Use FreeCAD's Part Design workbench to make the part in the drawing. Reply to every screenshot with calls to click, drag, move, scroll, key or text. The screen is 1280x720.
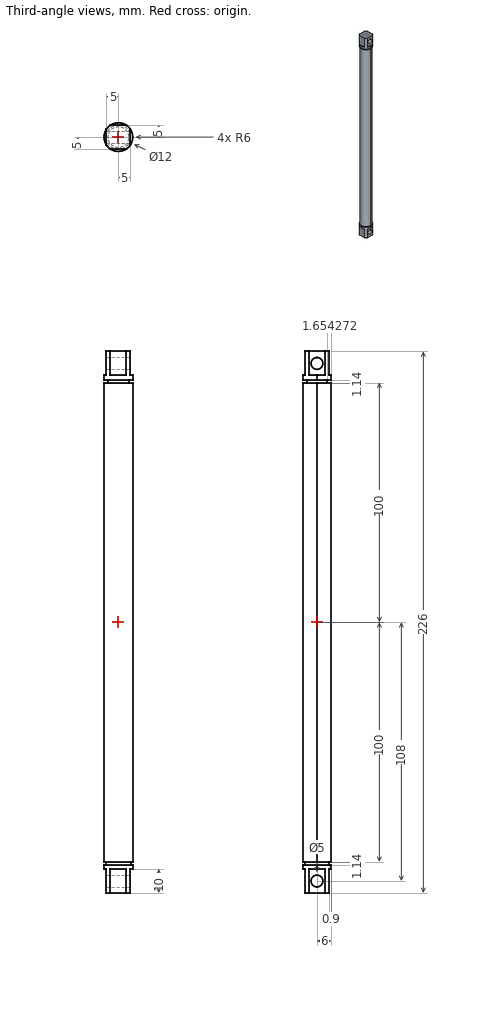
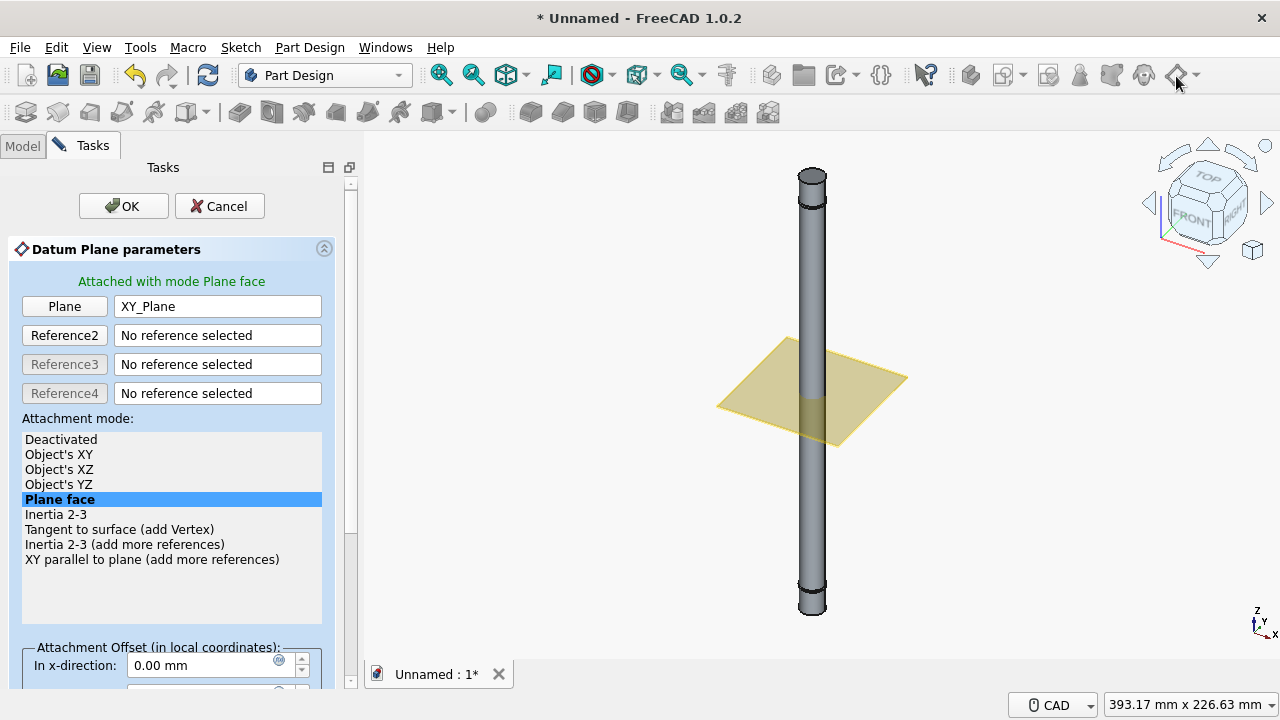
scroll(351, 432, down, 2)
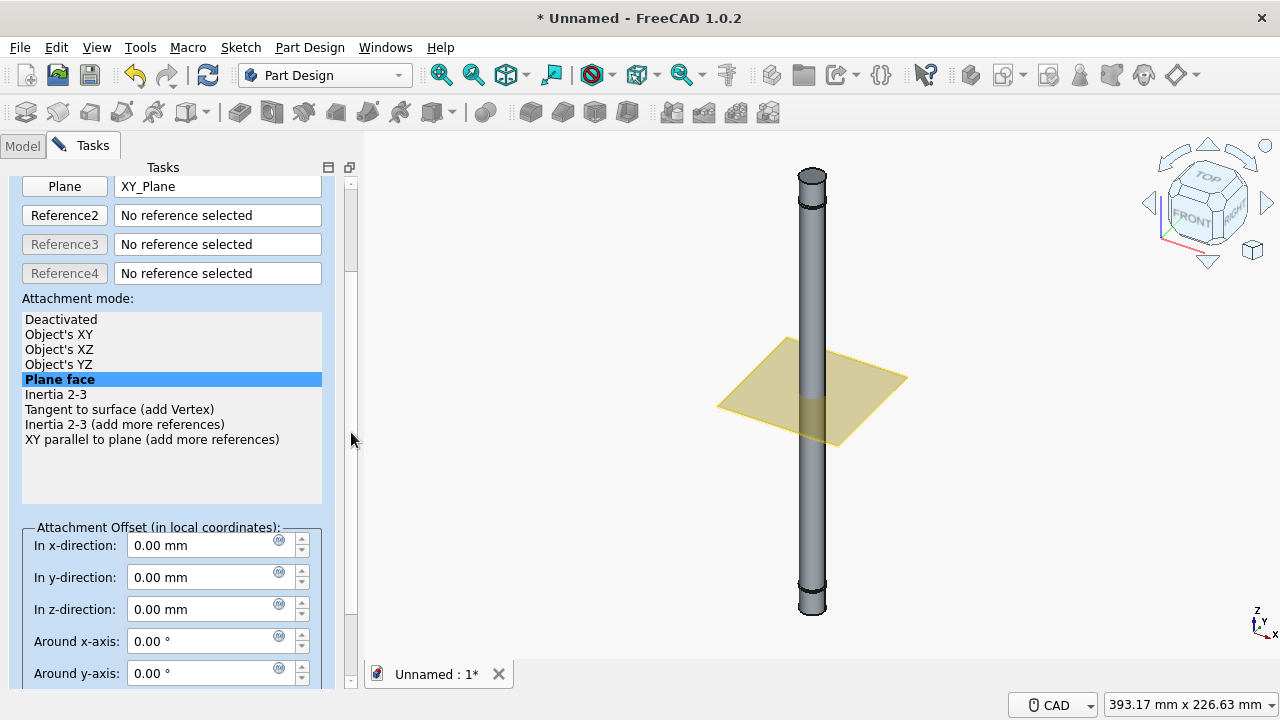
triple_click(210, 609)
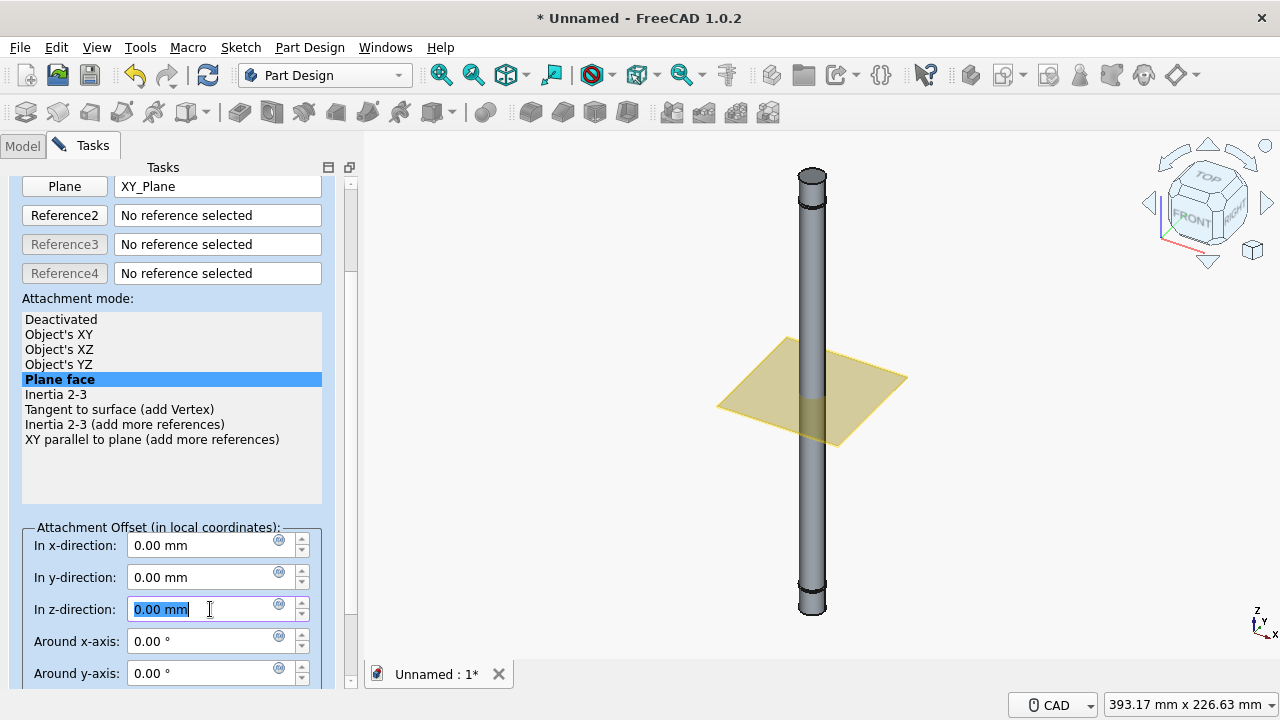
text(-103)
key(Tab)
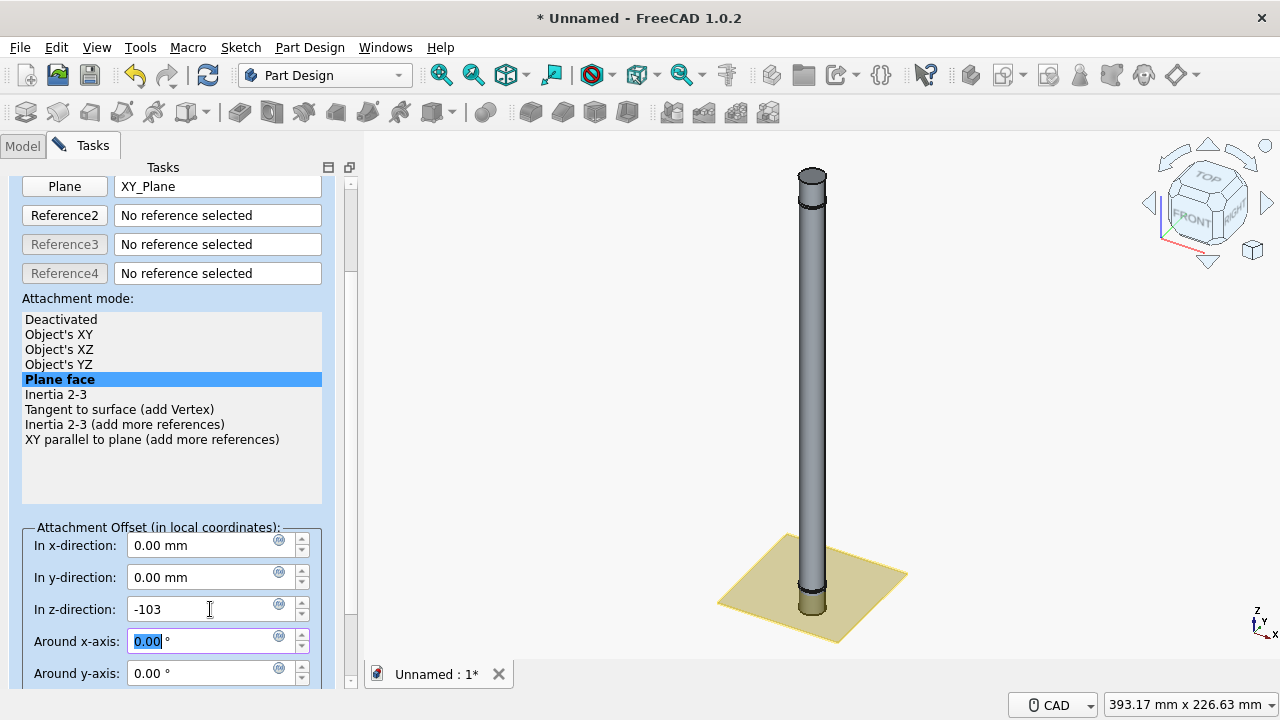
scroll(351, 432, up, 3)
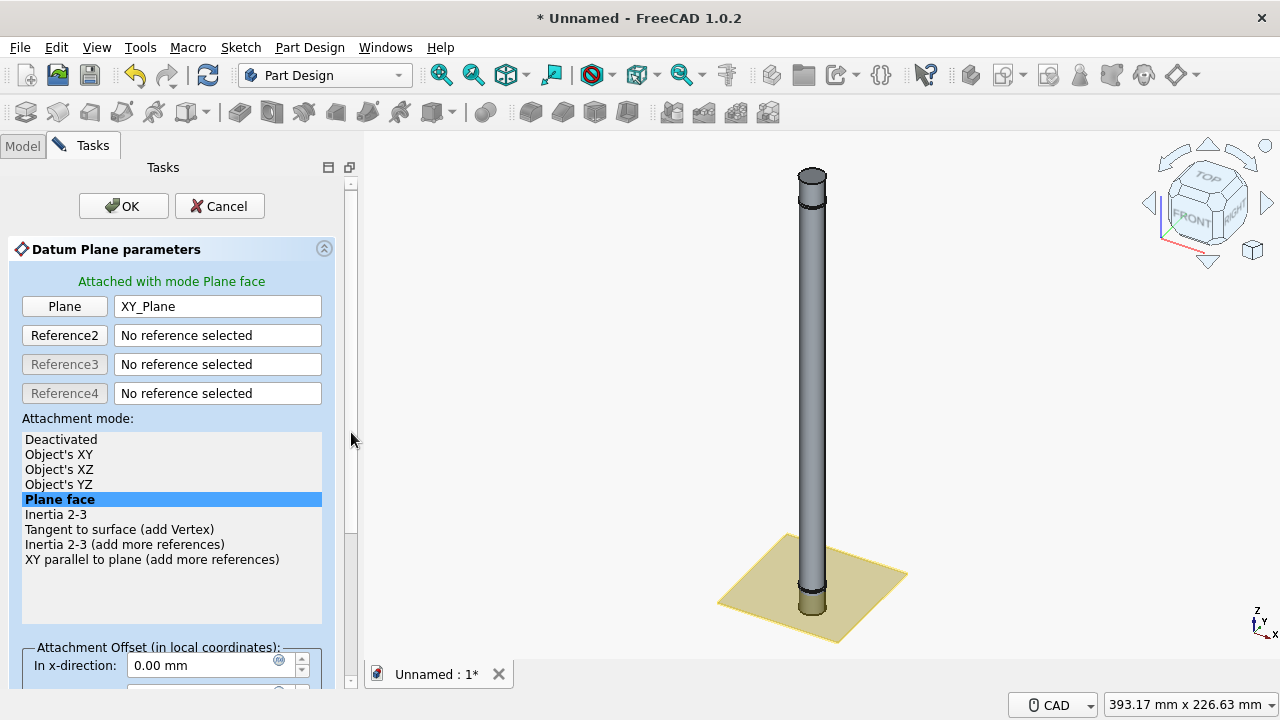
click(124, 206)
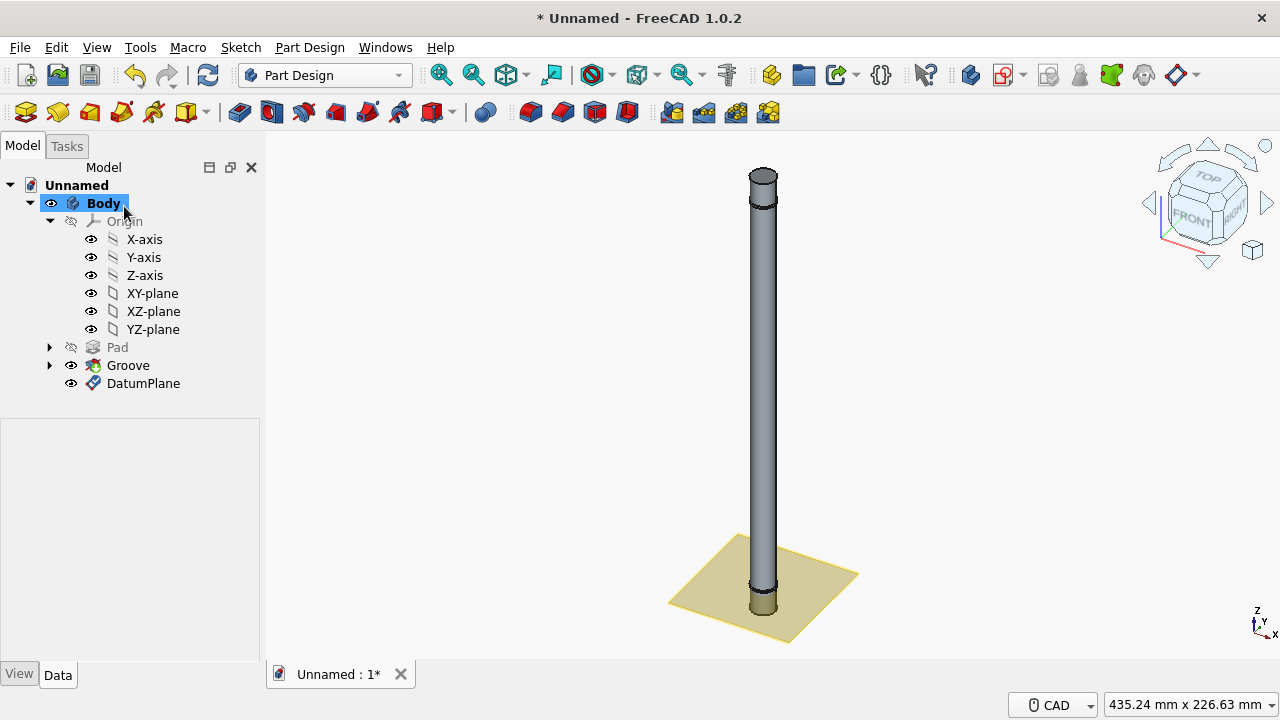
click(116, 383)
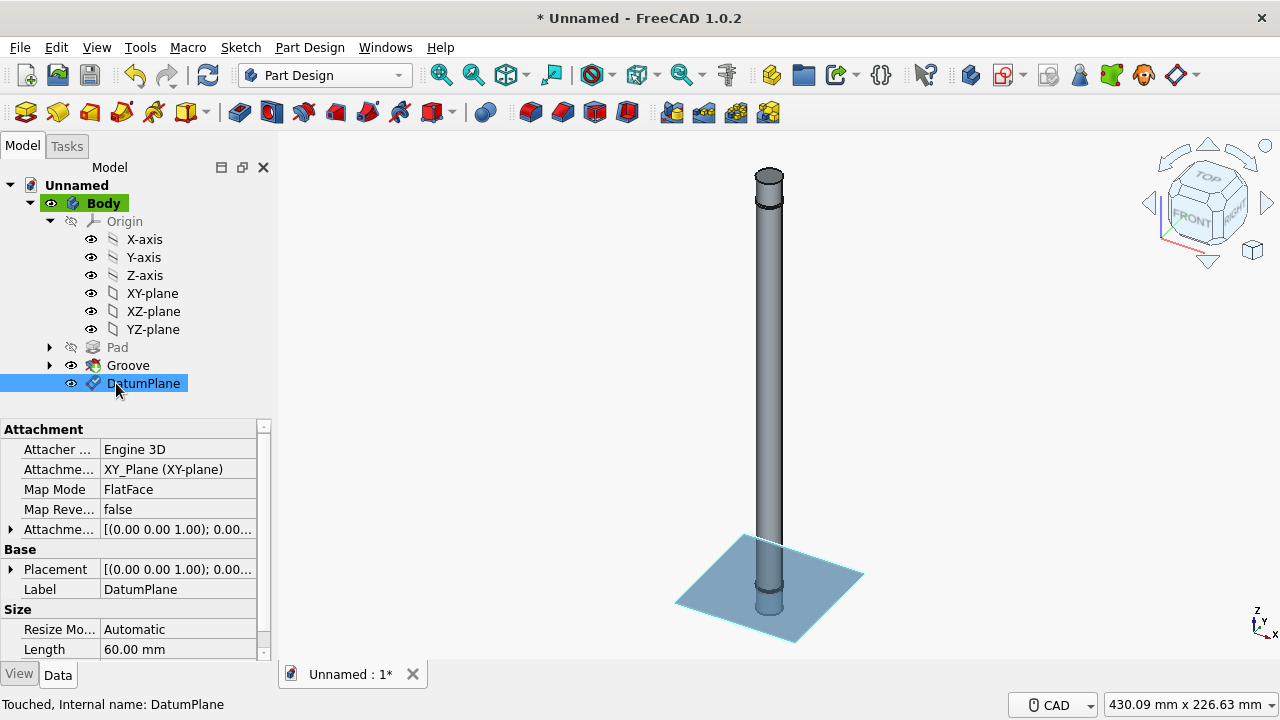
click(1004, 76)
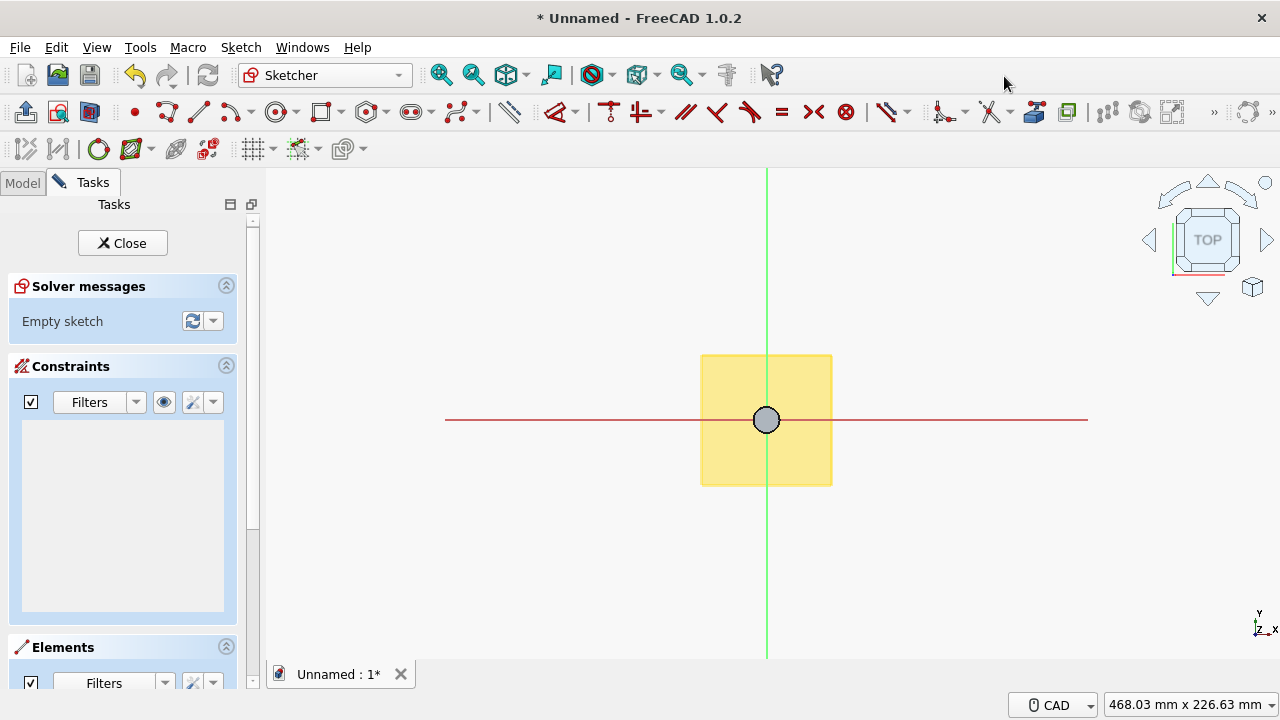
click(90, 112)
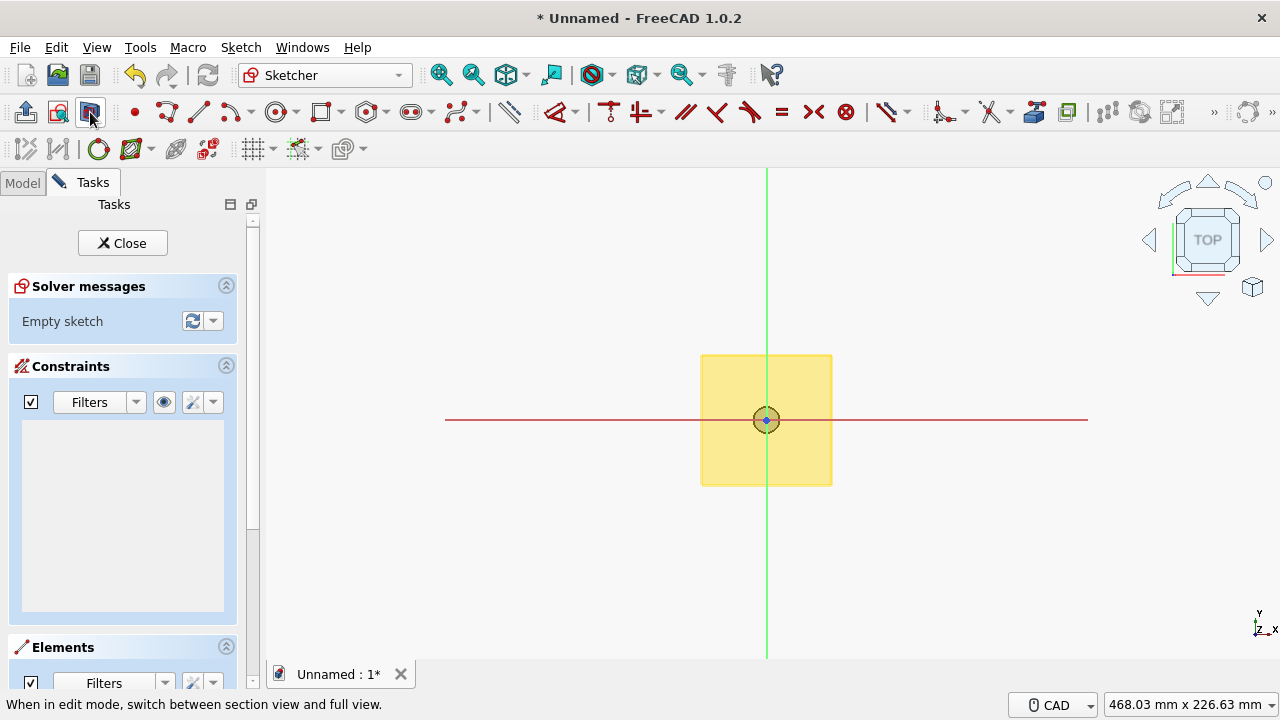
scroll(773, 421, up, 12)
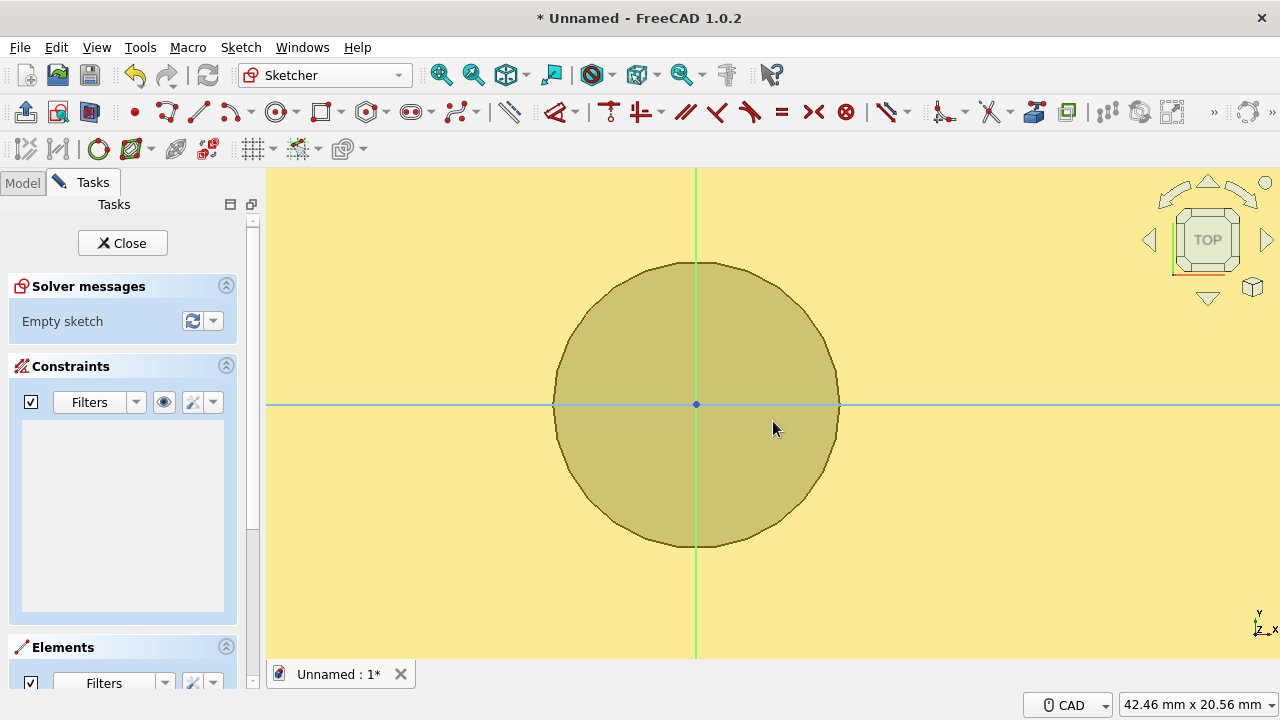
click(200, 112)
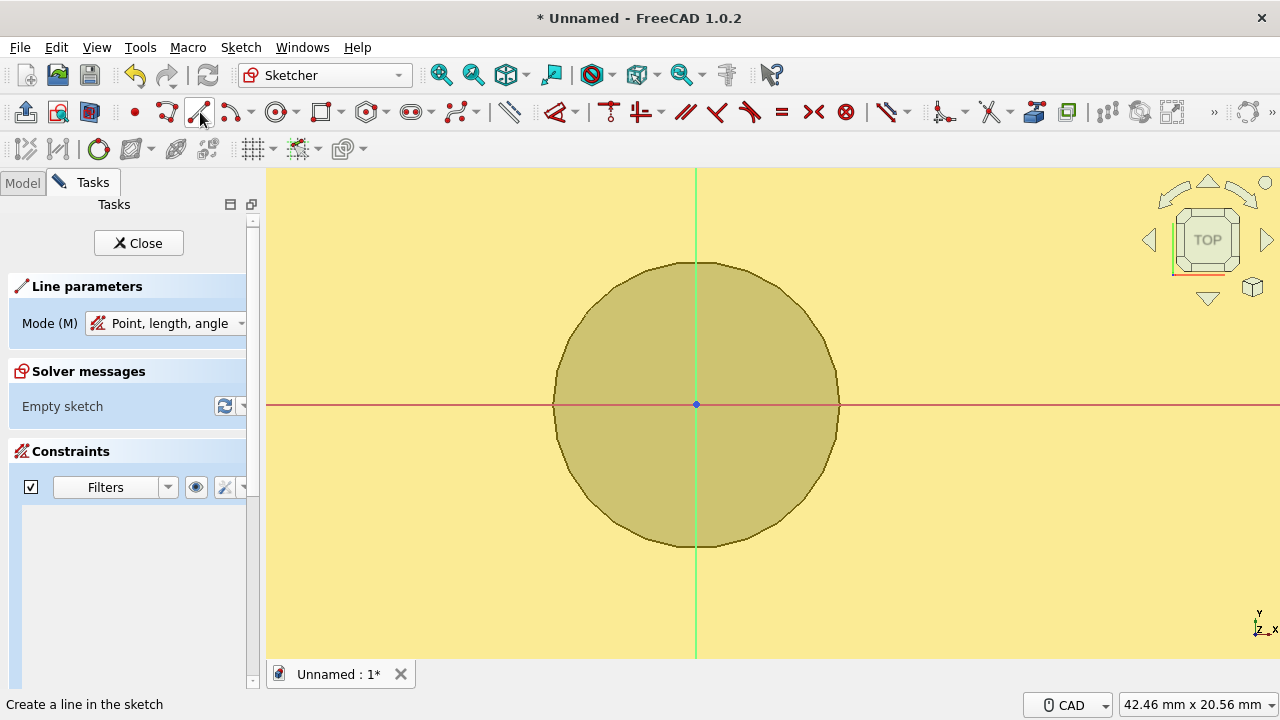
click(816, 484)
click(816, 326)